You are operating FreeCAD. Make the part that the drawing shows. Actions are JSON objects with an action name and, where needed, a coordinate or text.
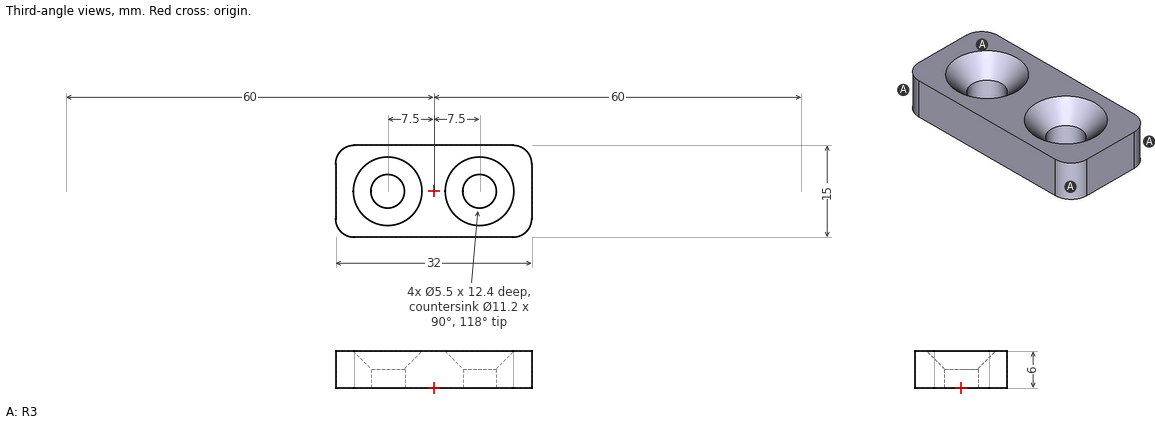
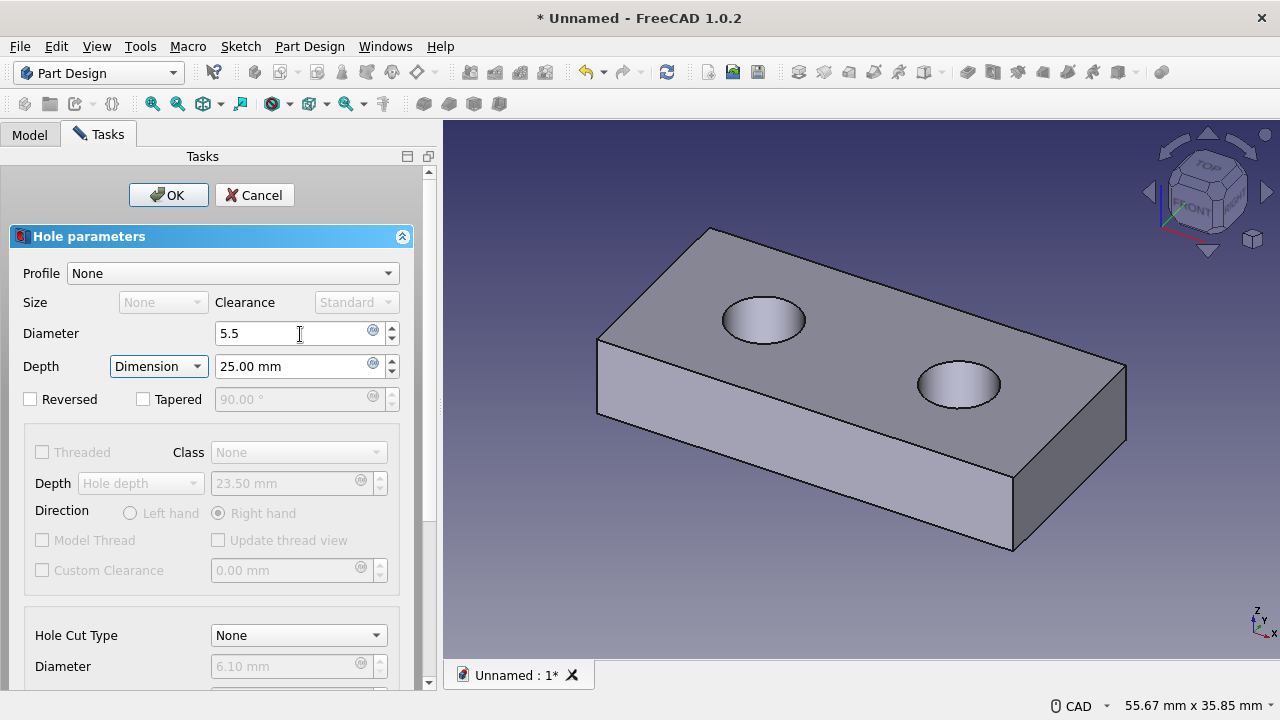
{"action": "triple_click", "coordinate": [300, 366]}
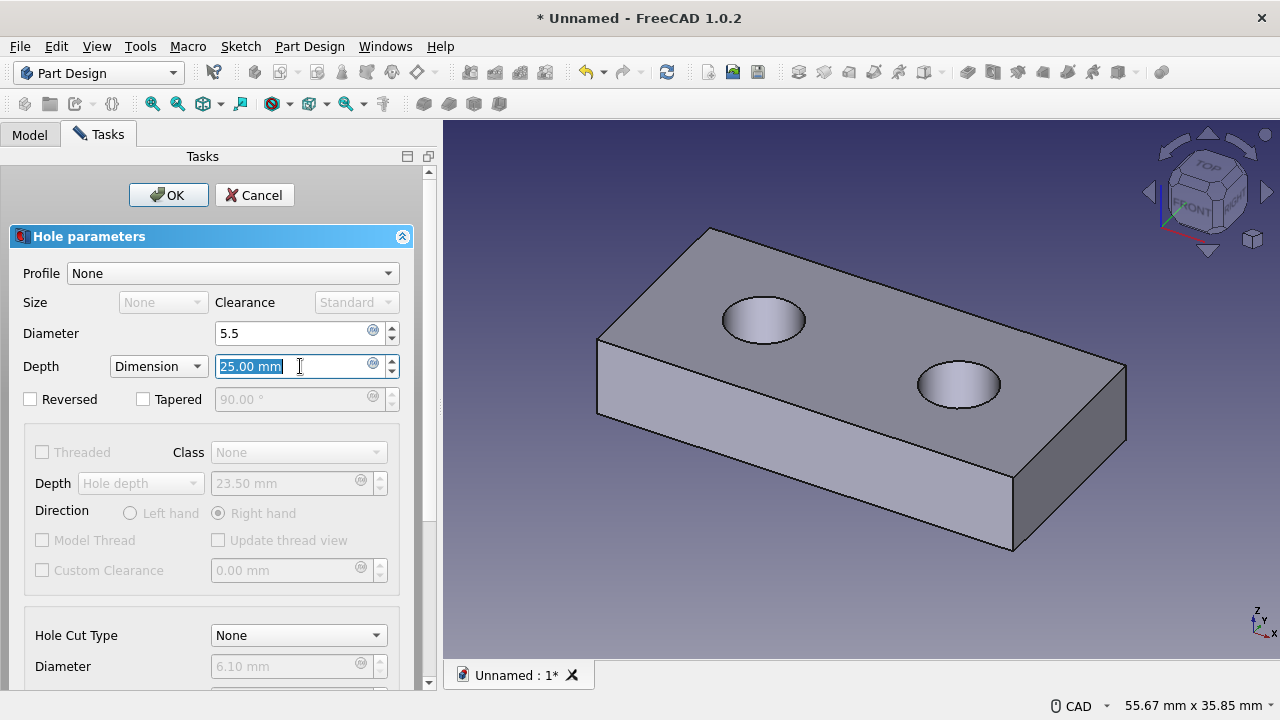
{"action": "type", "text": "12.4"}
{"action": "key", "text": "Tab"}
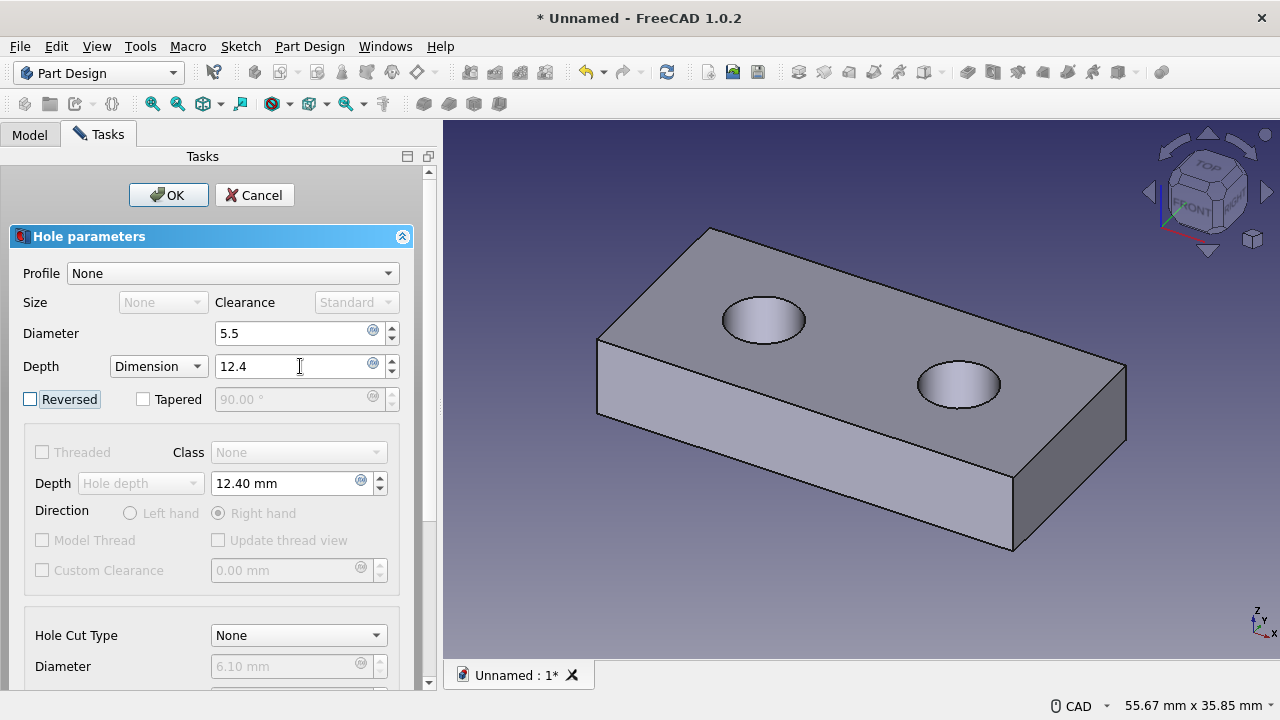
{"action": "left_click", "coordinate": [300, 636]}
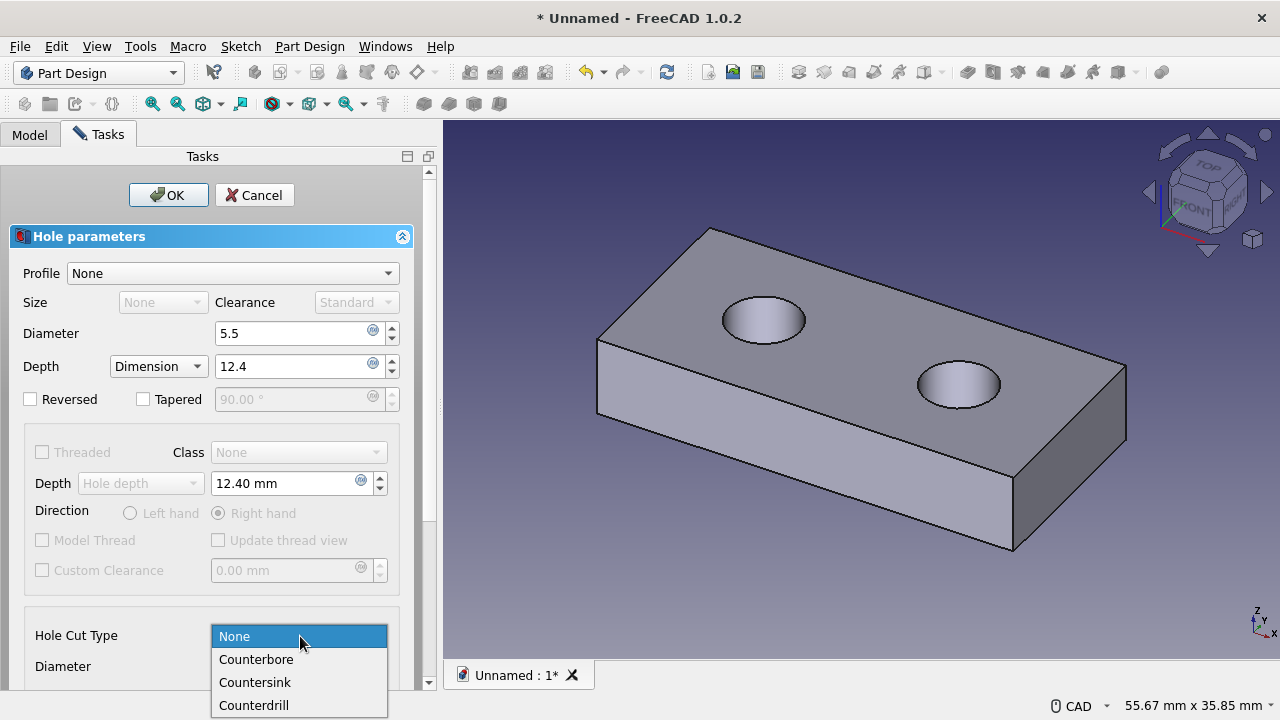
{"action": "left_click", "coordinate": [298, 682]}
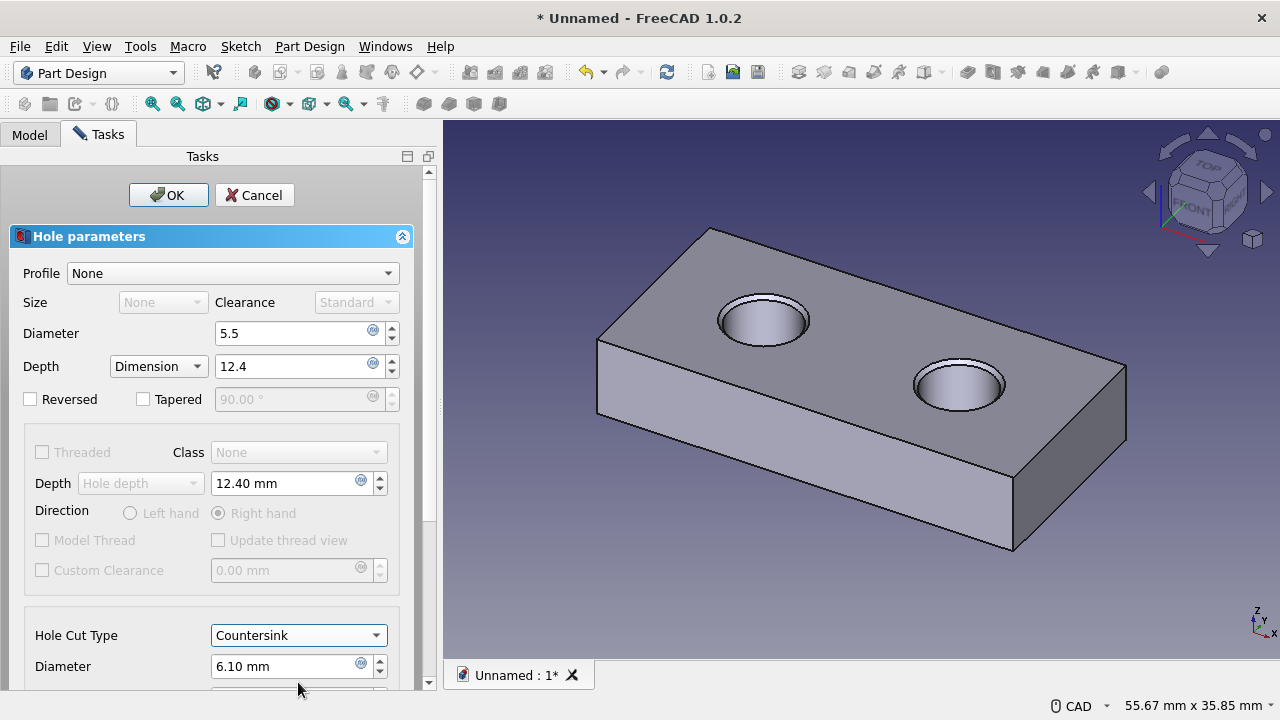
{"action": "triple_click", "coordinate": [292, 666]}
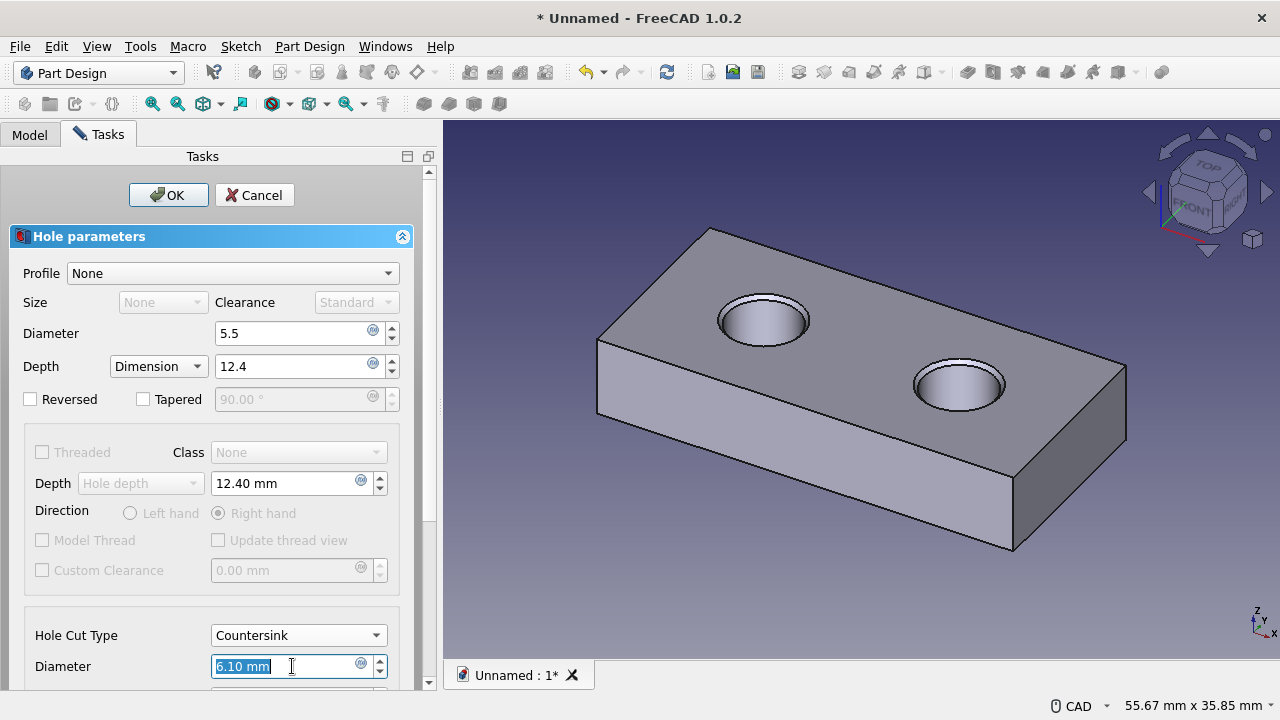
{"action": "type", "text": "11.2"}
{"action": "key", "text": "Tab"}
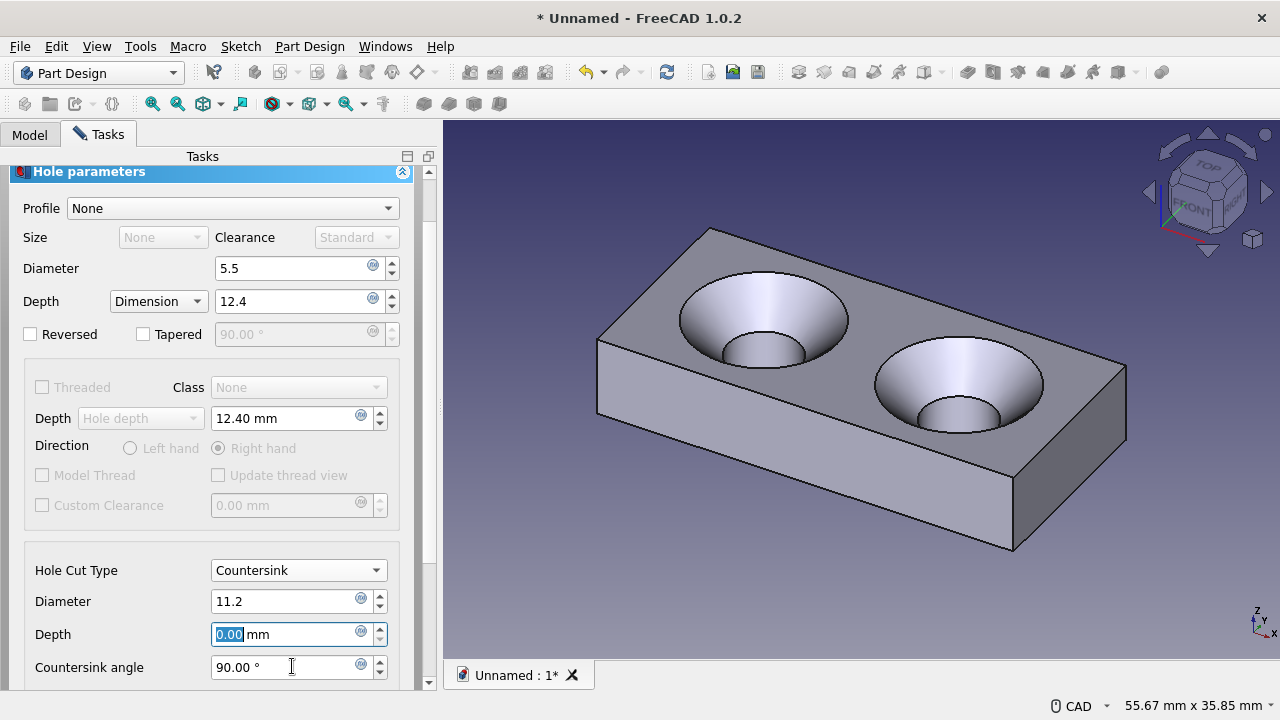
{"action": "scroll", "coordinate": [429, 428], "scroll_direction": "up", "scroll_amount": 2}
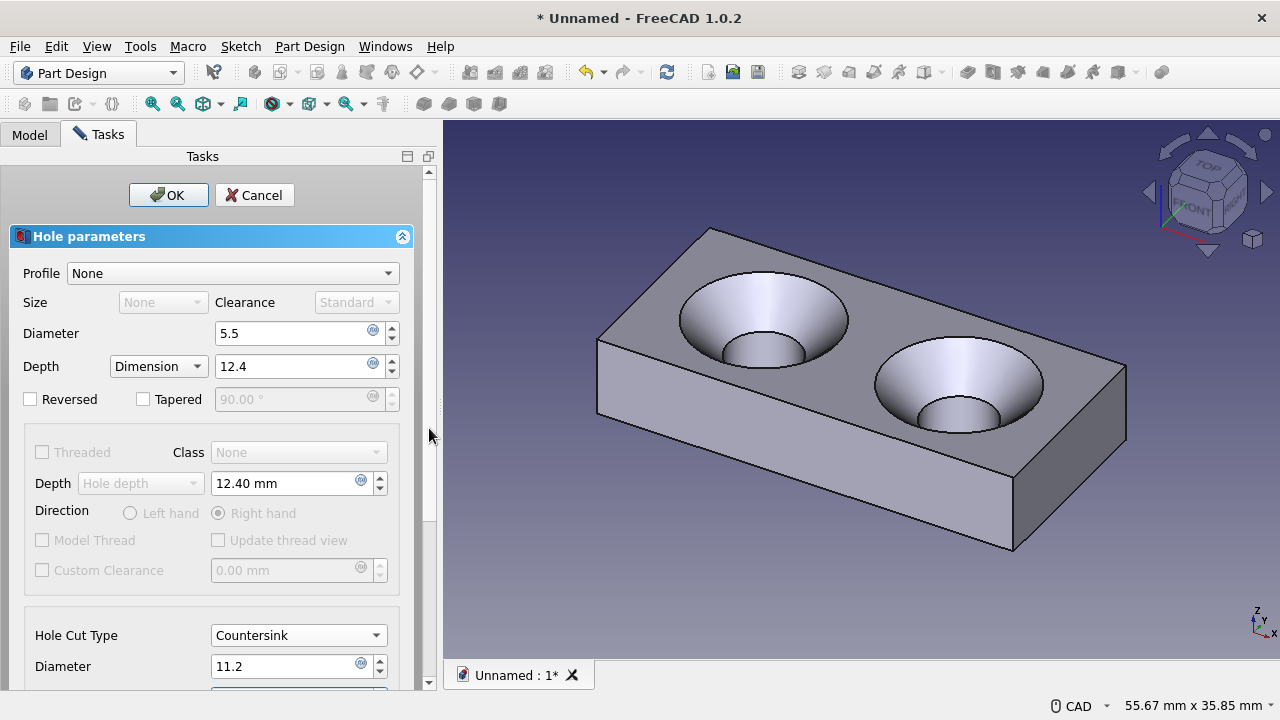
{"action": "left_click", "coordinate": [169, 195]}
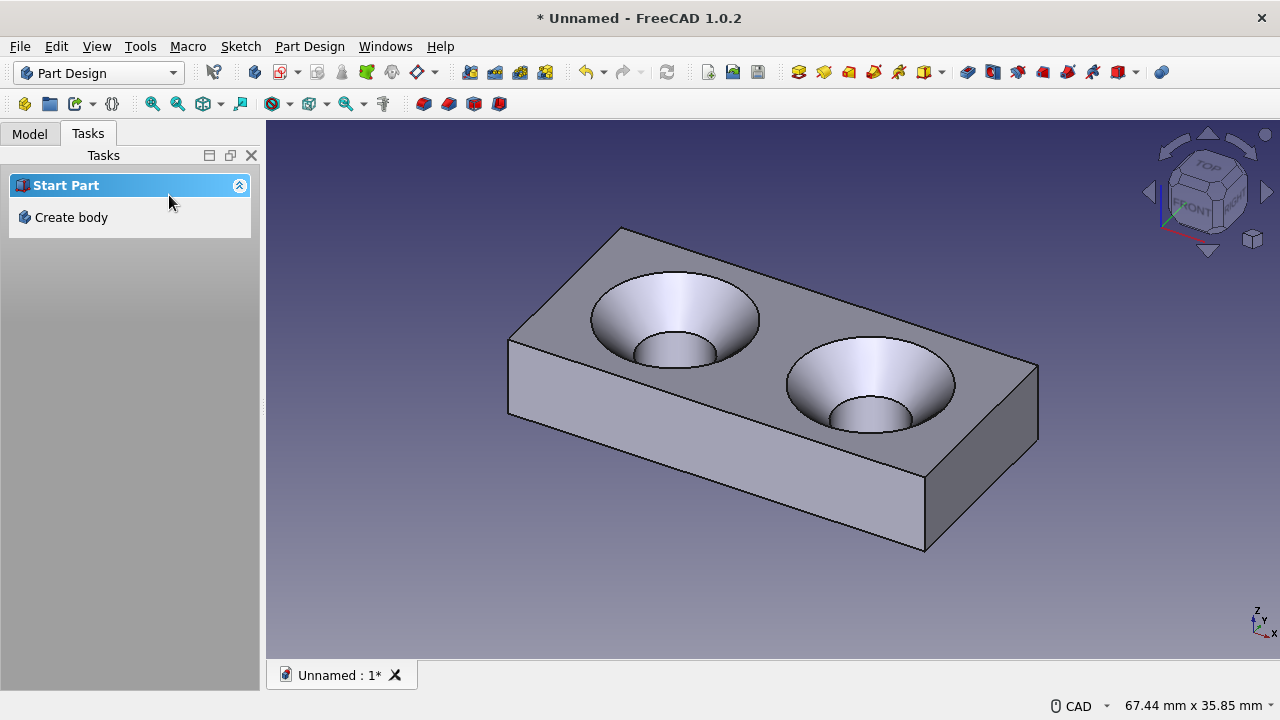
{"action": "left_click", "coordinate": [925, 514]}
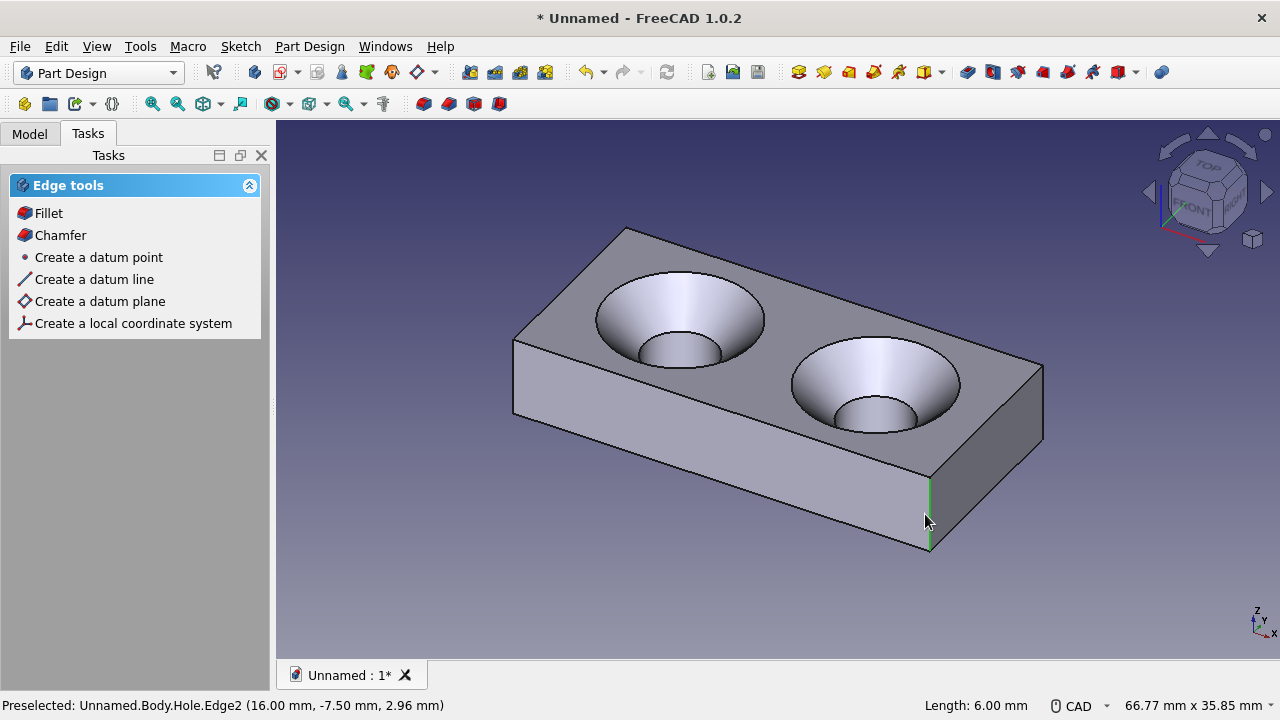
{"action": "key", "text": "0"}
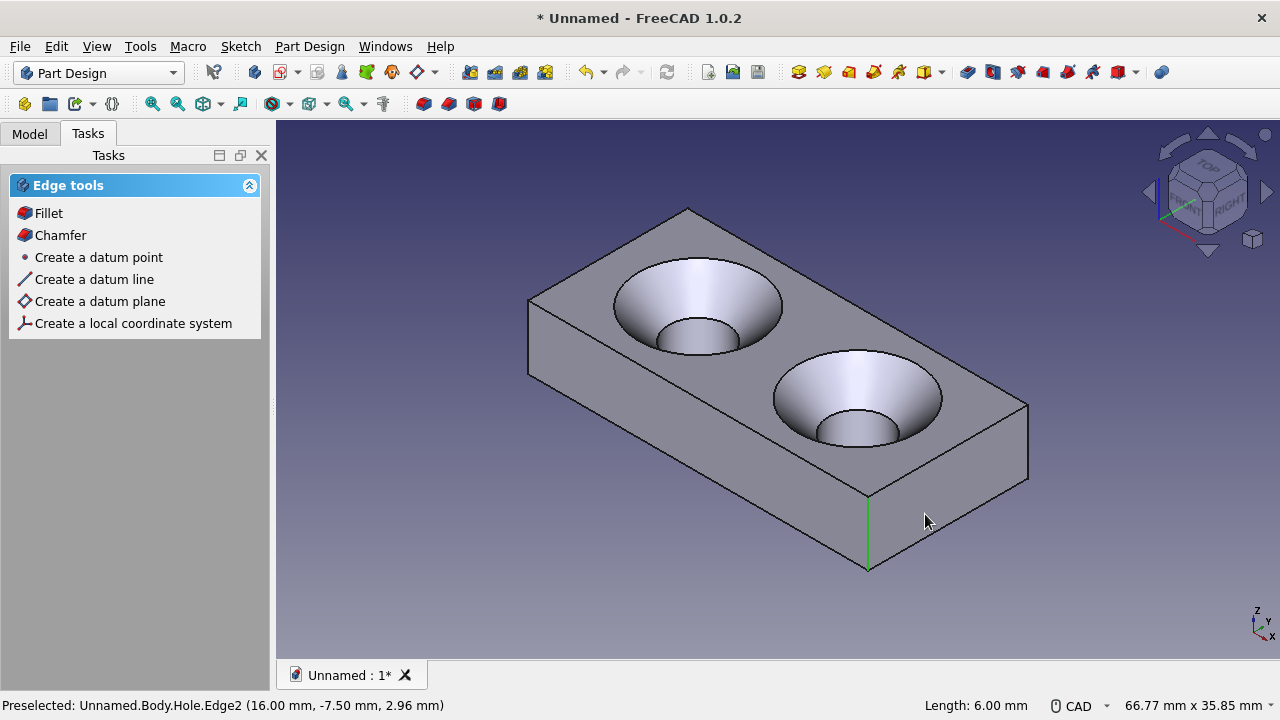
{"action": "key", "text": "2"}